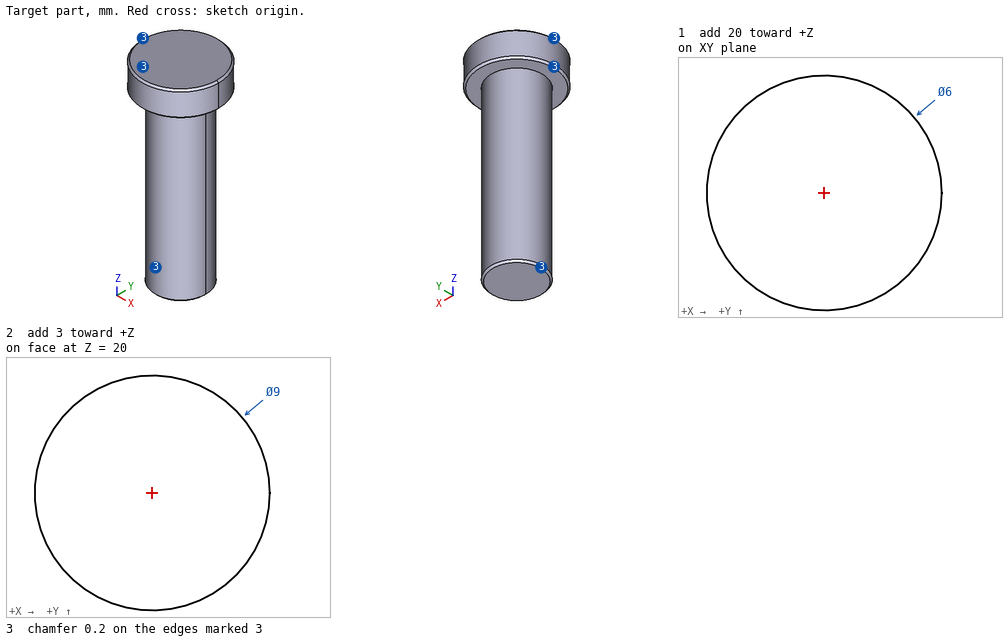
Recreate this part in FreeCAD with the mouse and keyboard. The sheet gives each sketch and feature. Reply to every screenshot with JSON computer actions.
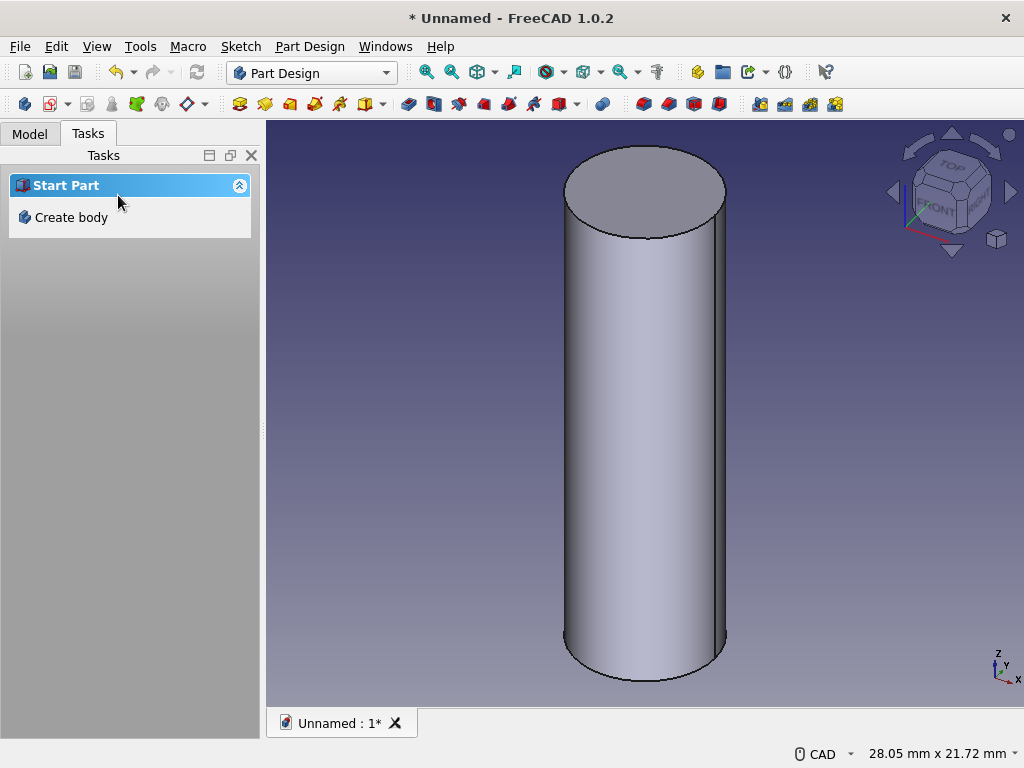
{"action": "left_click", "coordinate": [645, 191]}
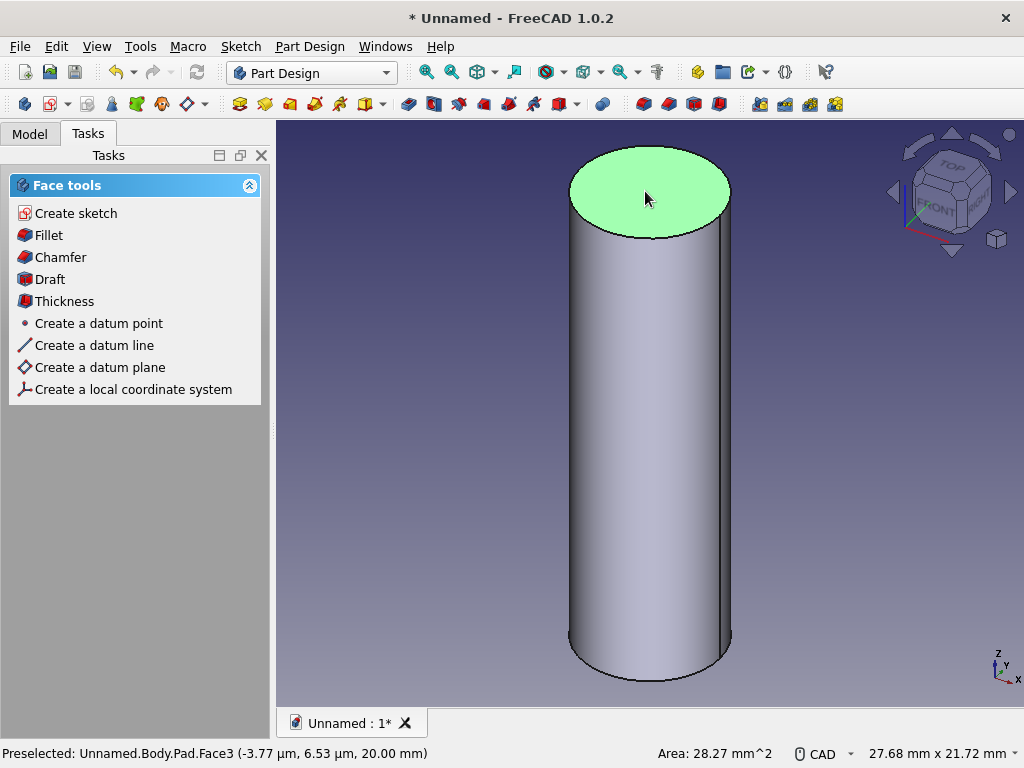
{"action": "left_click", "coordinate": [50, 104]}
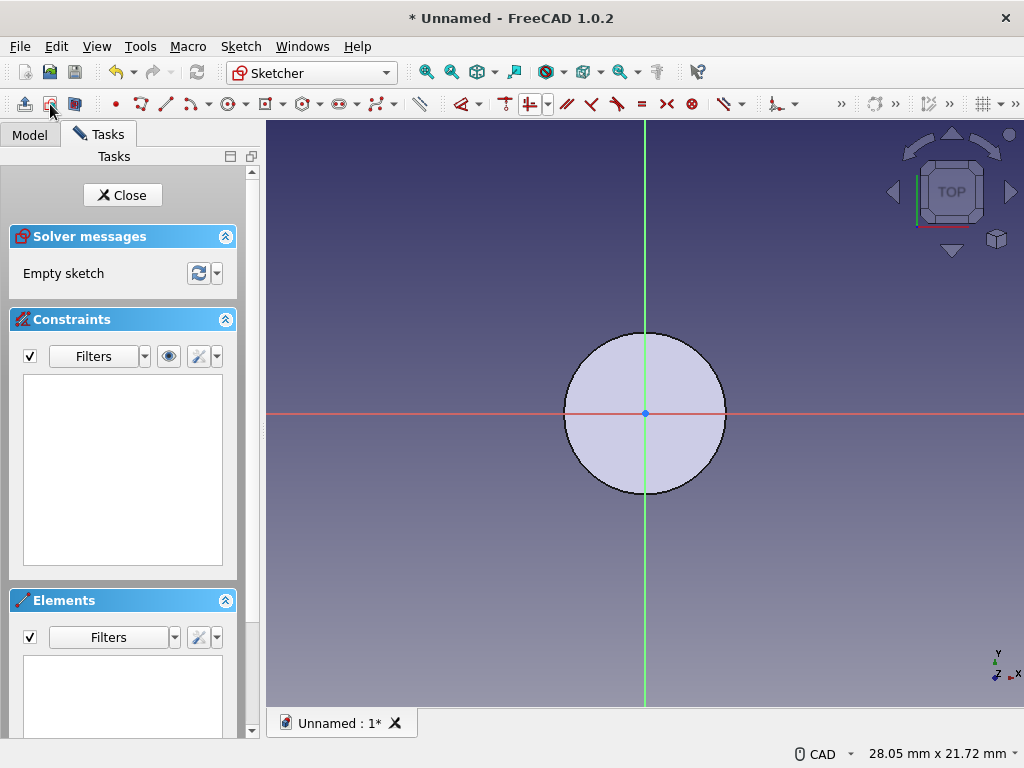
{"action": "scroll", "coordinate": [784, 413], "scroll_direction": "up", "scroll_amount": 2}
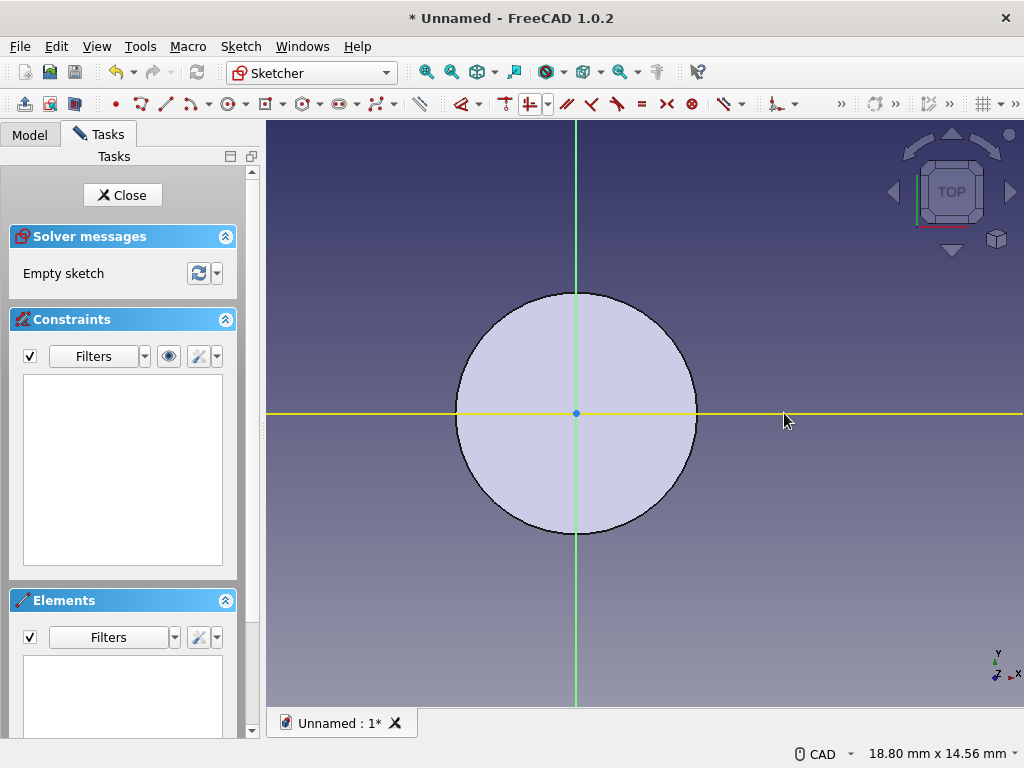
{"action": "key", "text": "g c"}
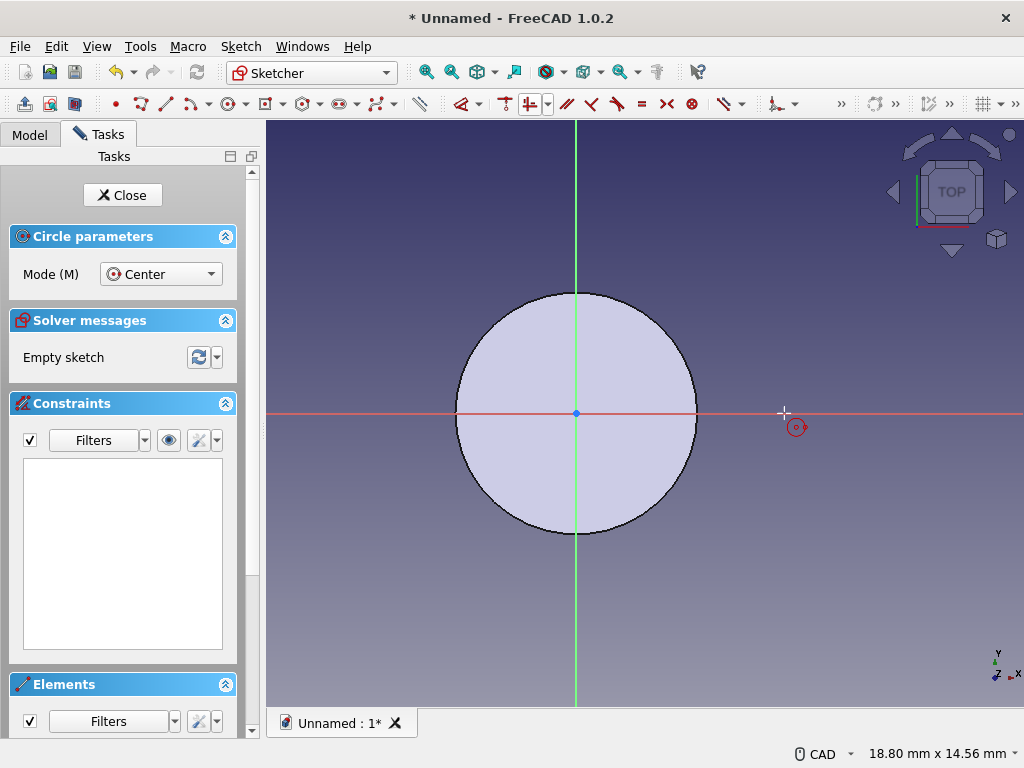
{"action": "left_click", "coordinate": [576, 414]}
{"action": "mouse_move", "coordinate": [705, 285]}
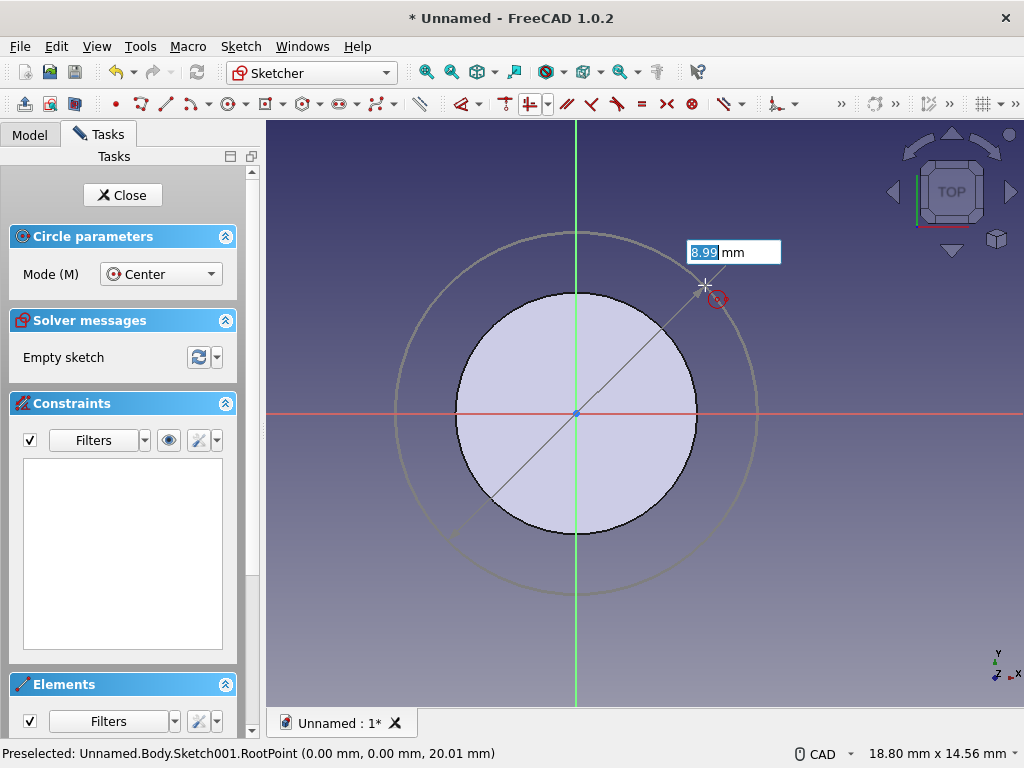
{"action": "type", "text": "9"}
{"action": "key", "text": "Return"}
{"action": "key", "text": "Escape"}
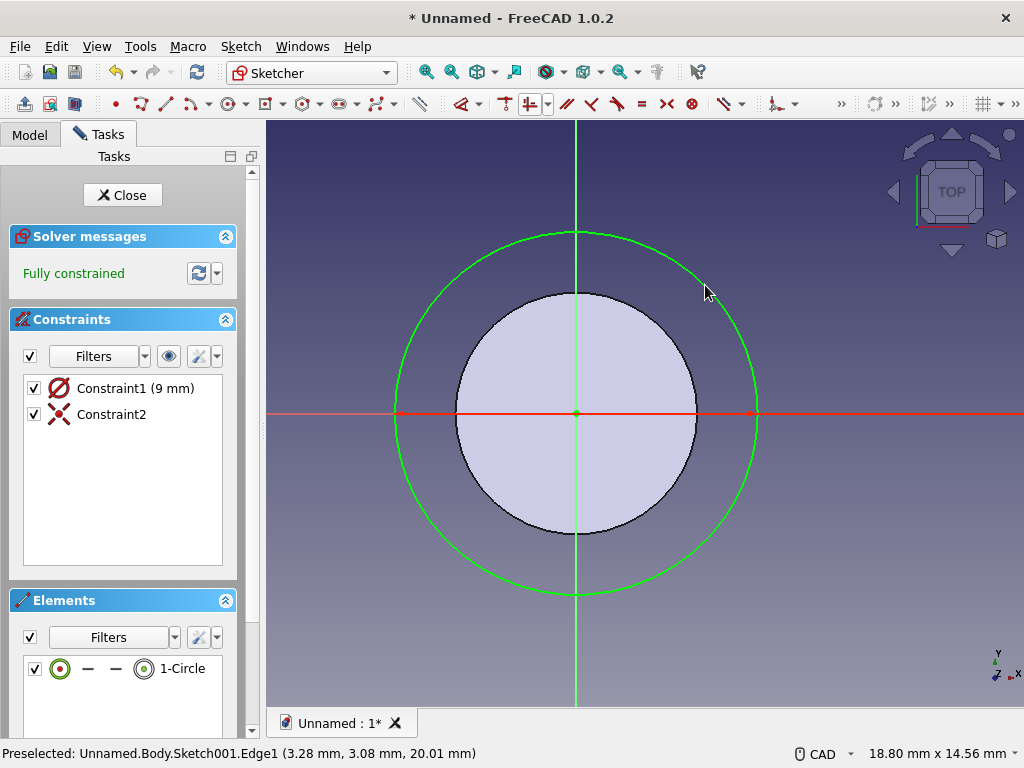
{"action": "left_click", "coordinate": [123, 195]}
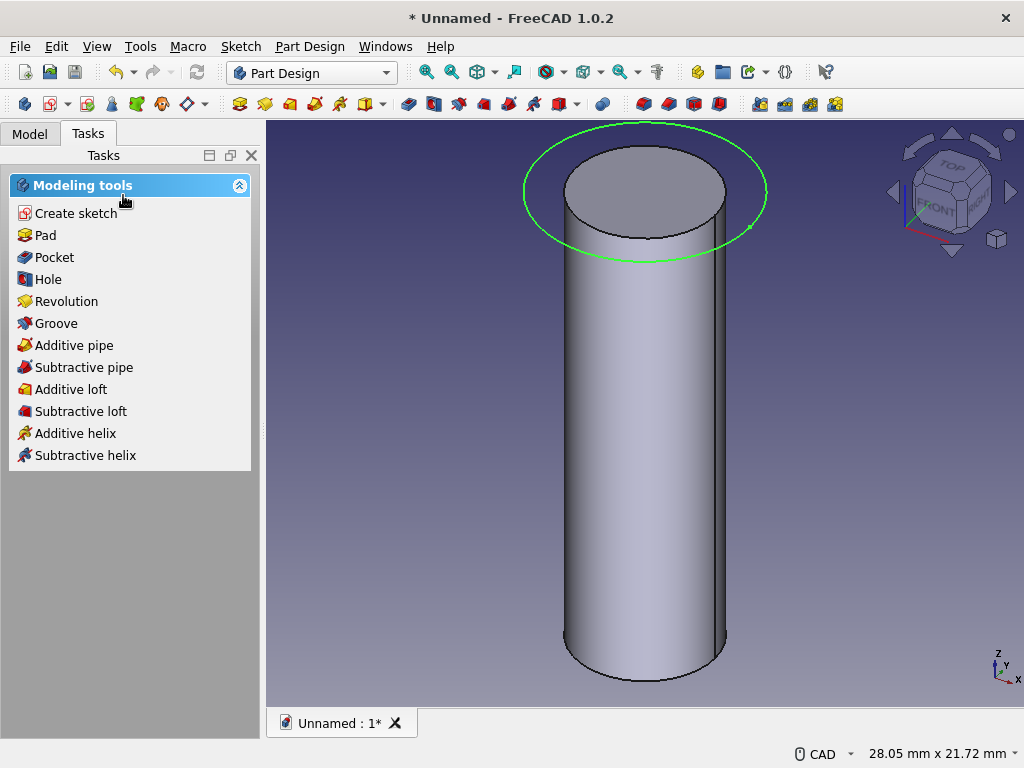
{"action": "left_click", "coordinate": [240, 104]}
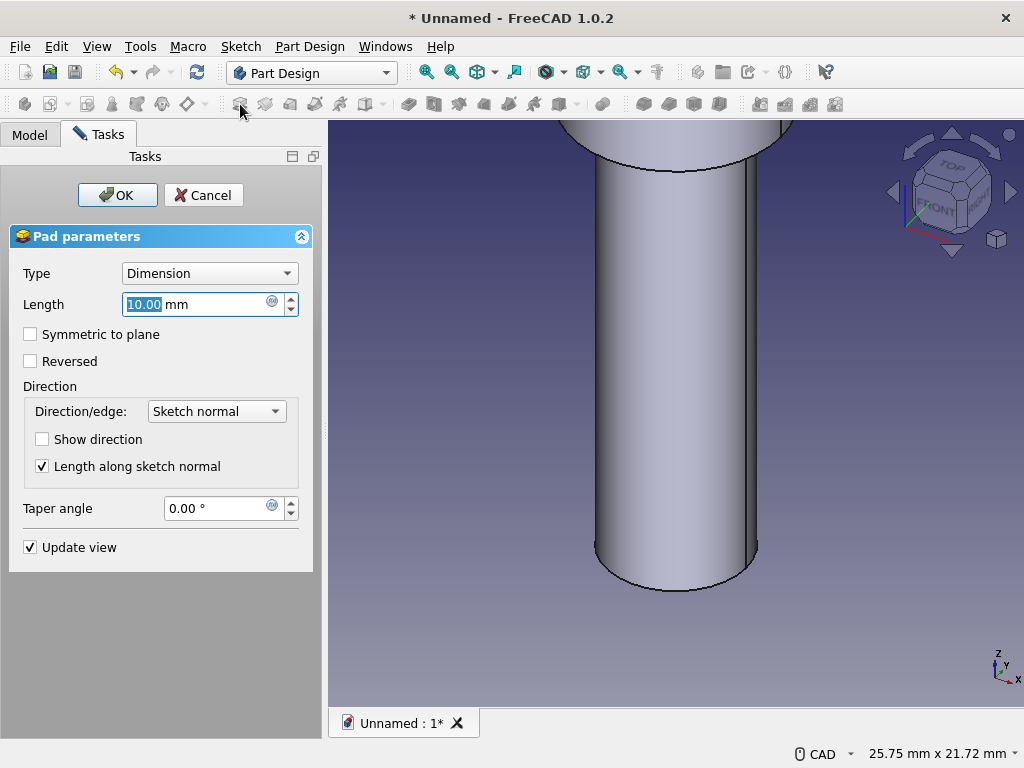
{"action": "type", "text": "3"}
{"action": "key", "text": "Tab"}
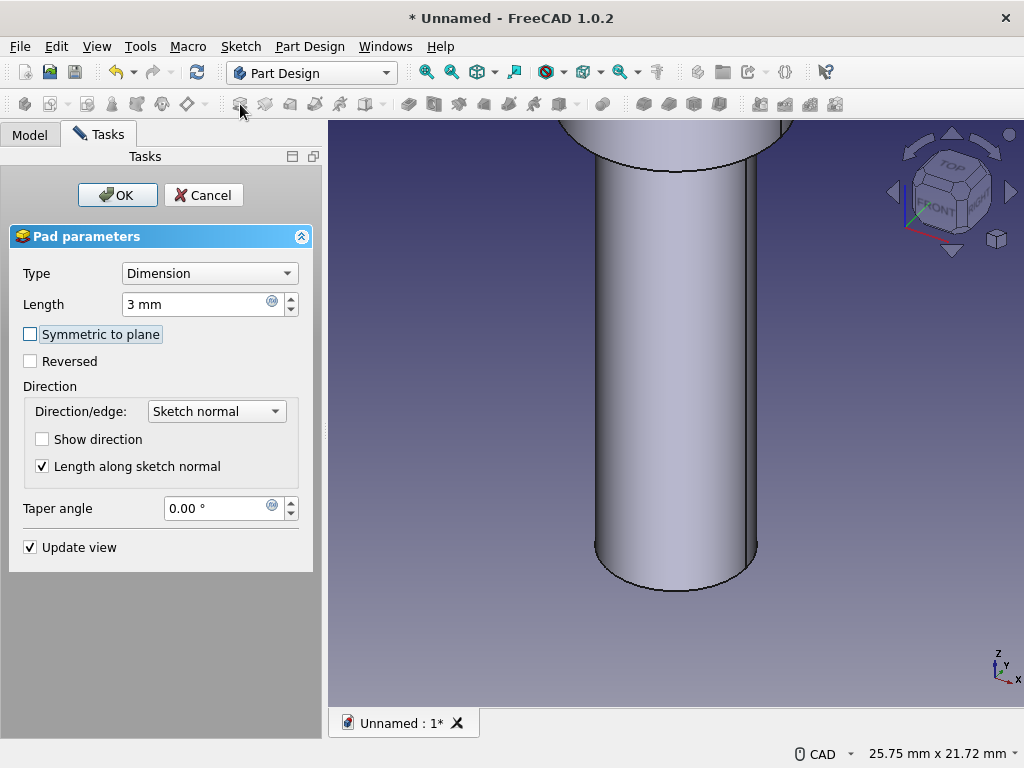
{"action": "left_click", "coordinate": [118, 195]}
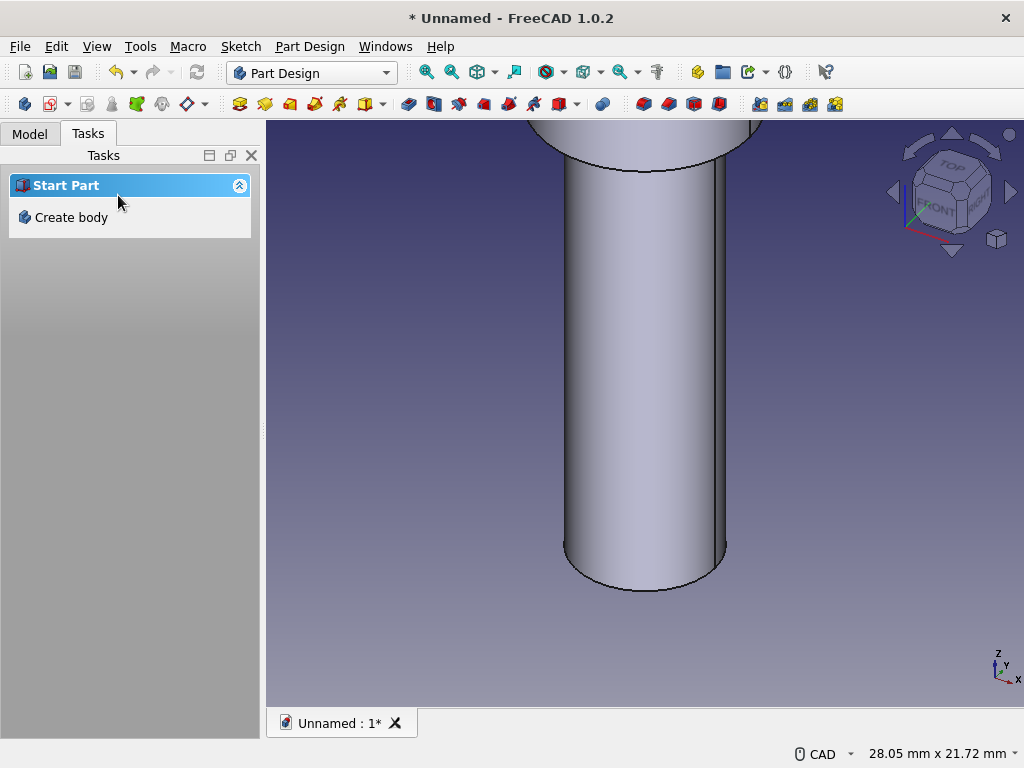
{"action": "key", "text": "v f"}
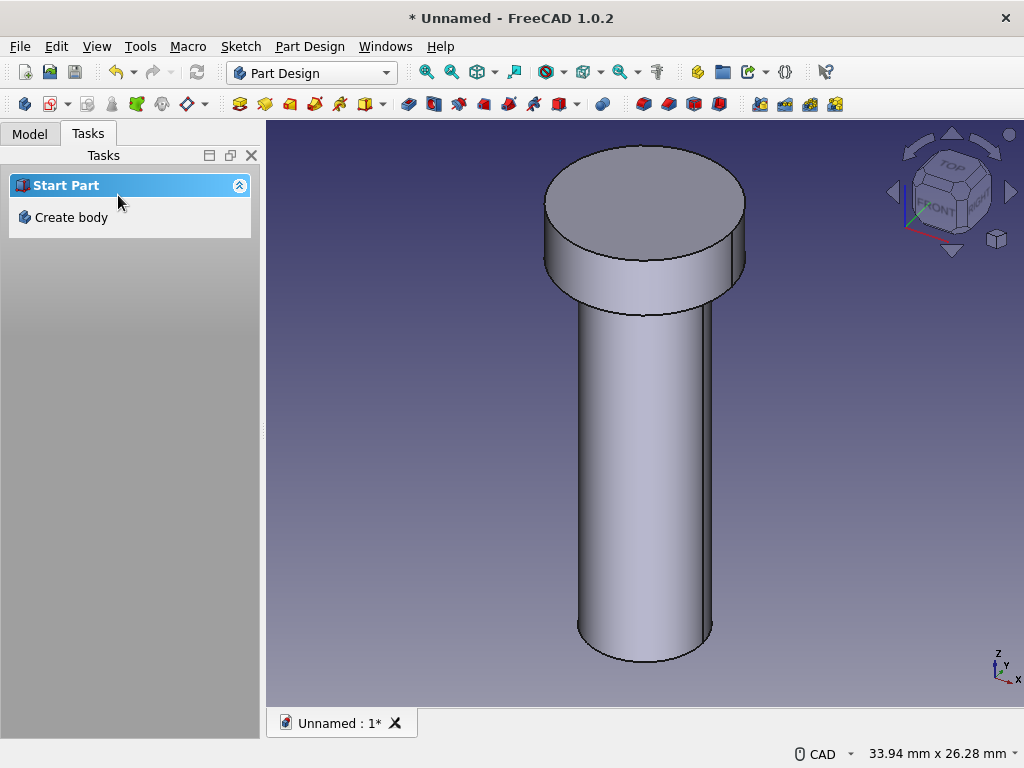
{"action": "left_click", "coordinate": [570, 296]}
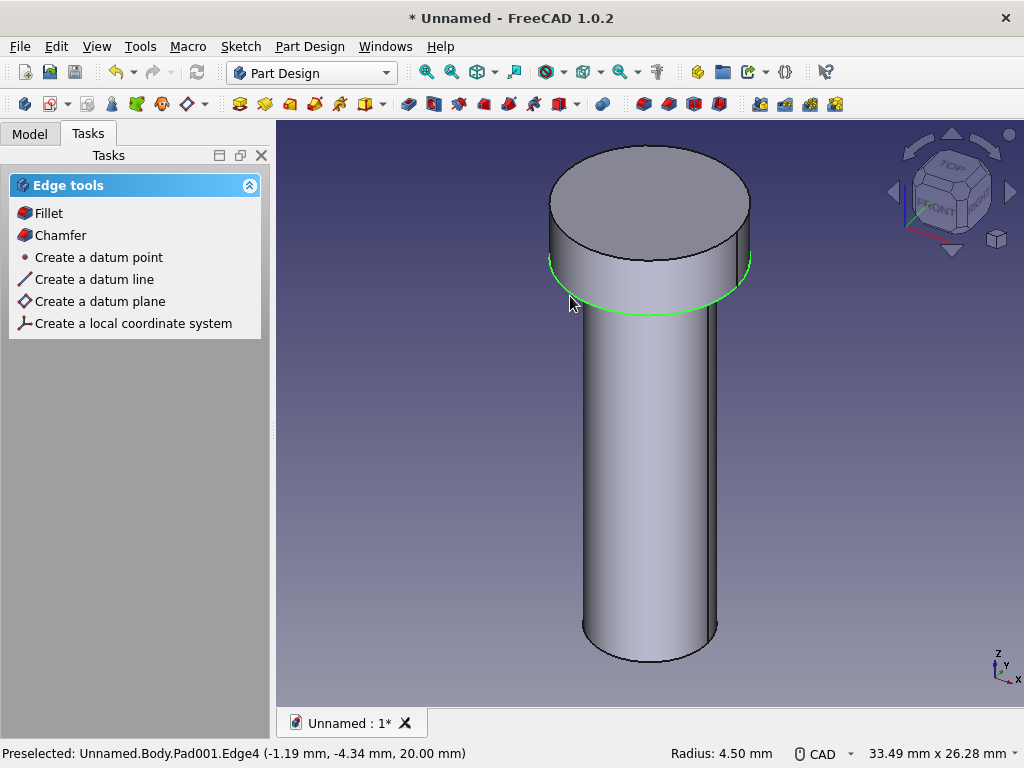
{"action": "left_click", "coordinate": [550, 208], "text": "ctrl"}